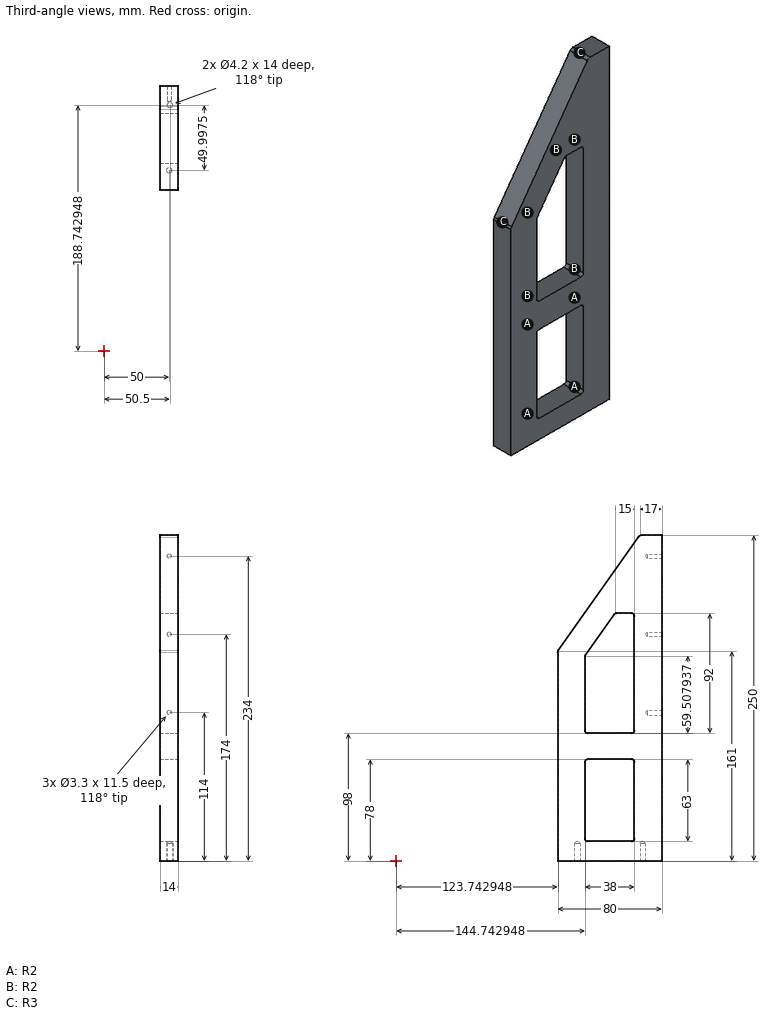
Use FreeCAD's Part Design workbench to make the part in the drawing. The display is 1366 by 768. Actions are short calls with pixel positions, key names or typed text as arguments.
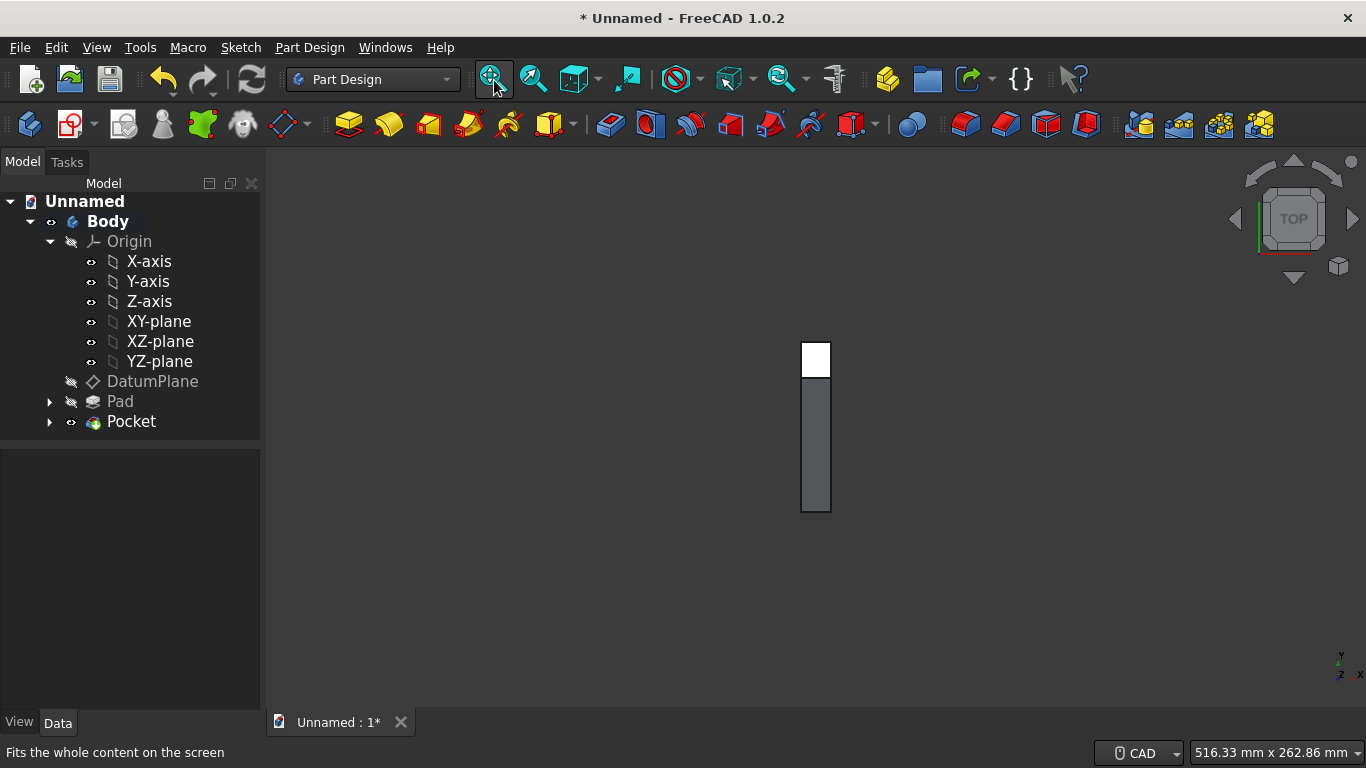
key(1)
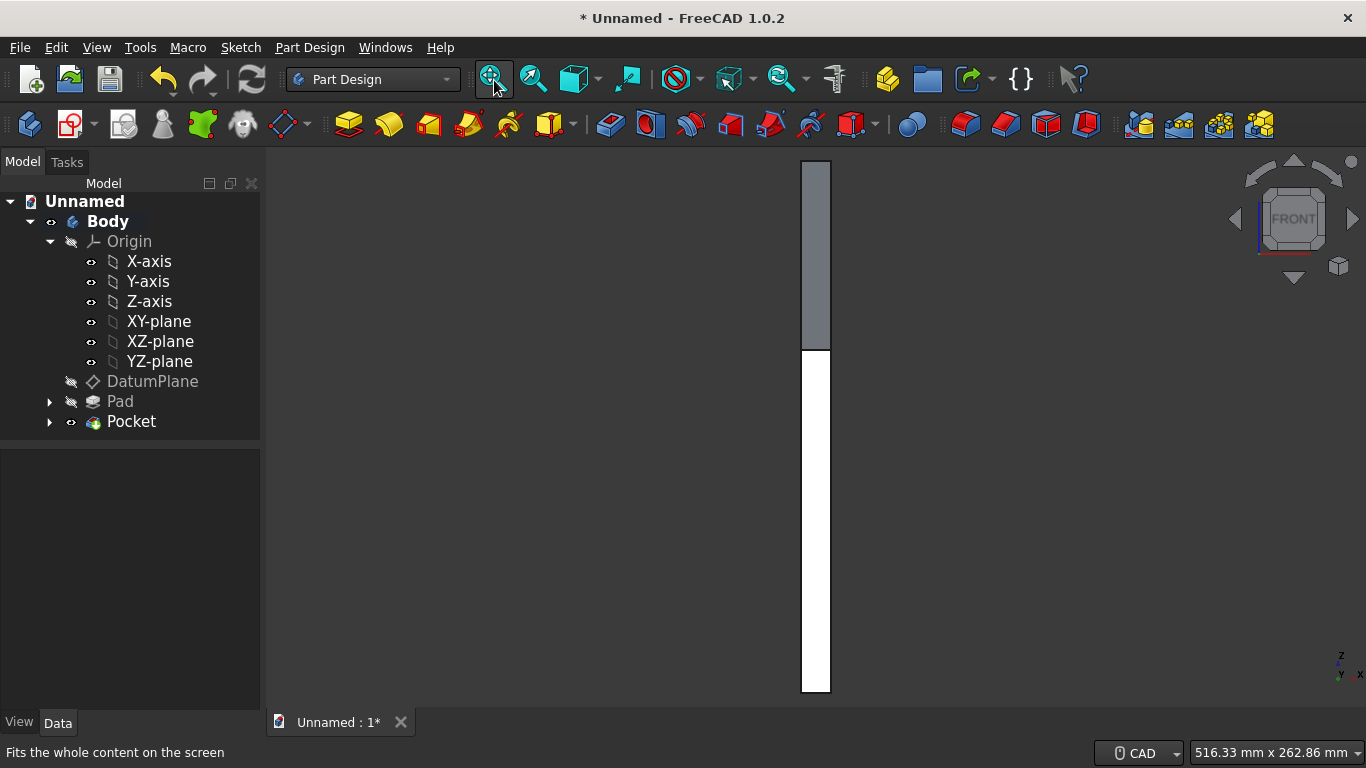
key(3)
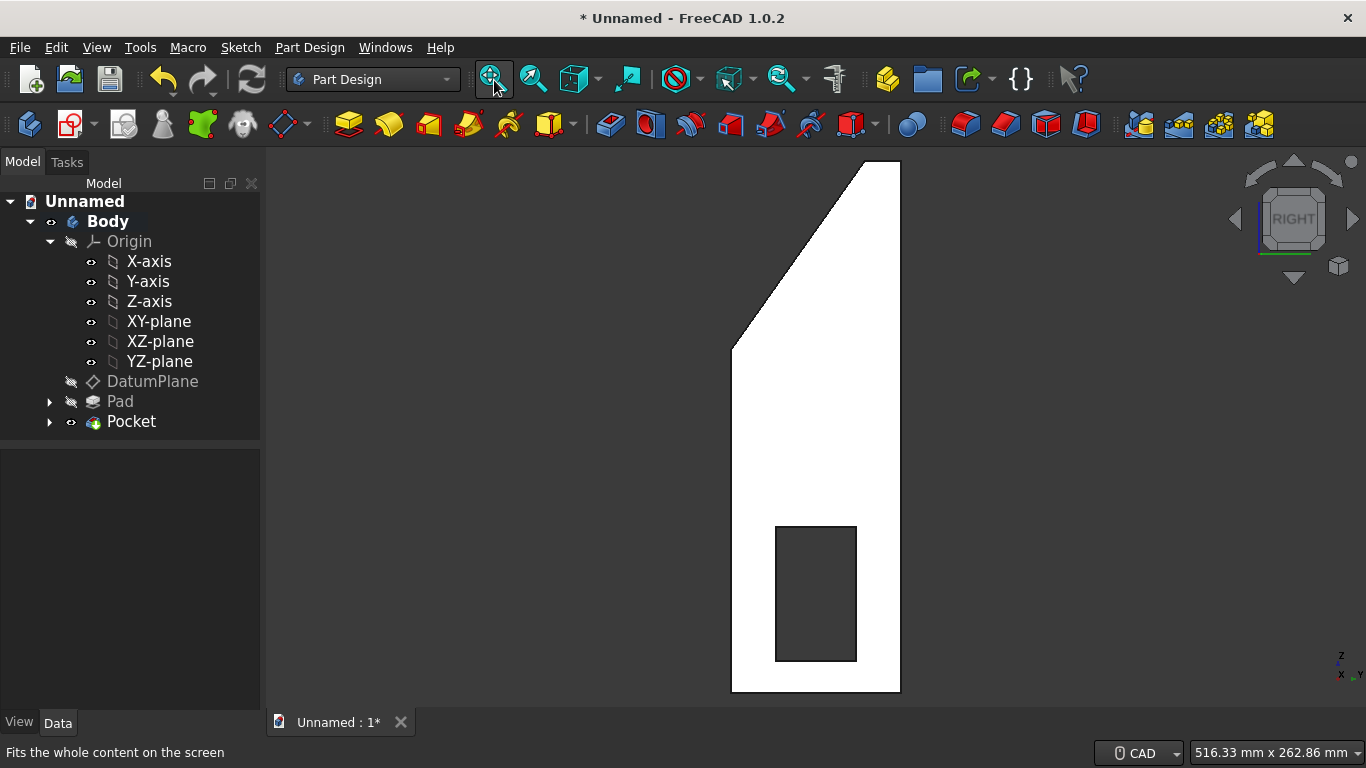
key(5)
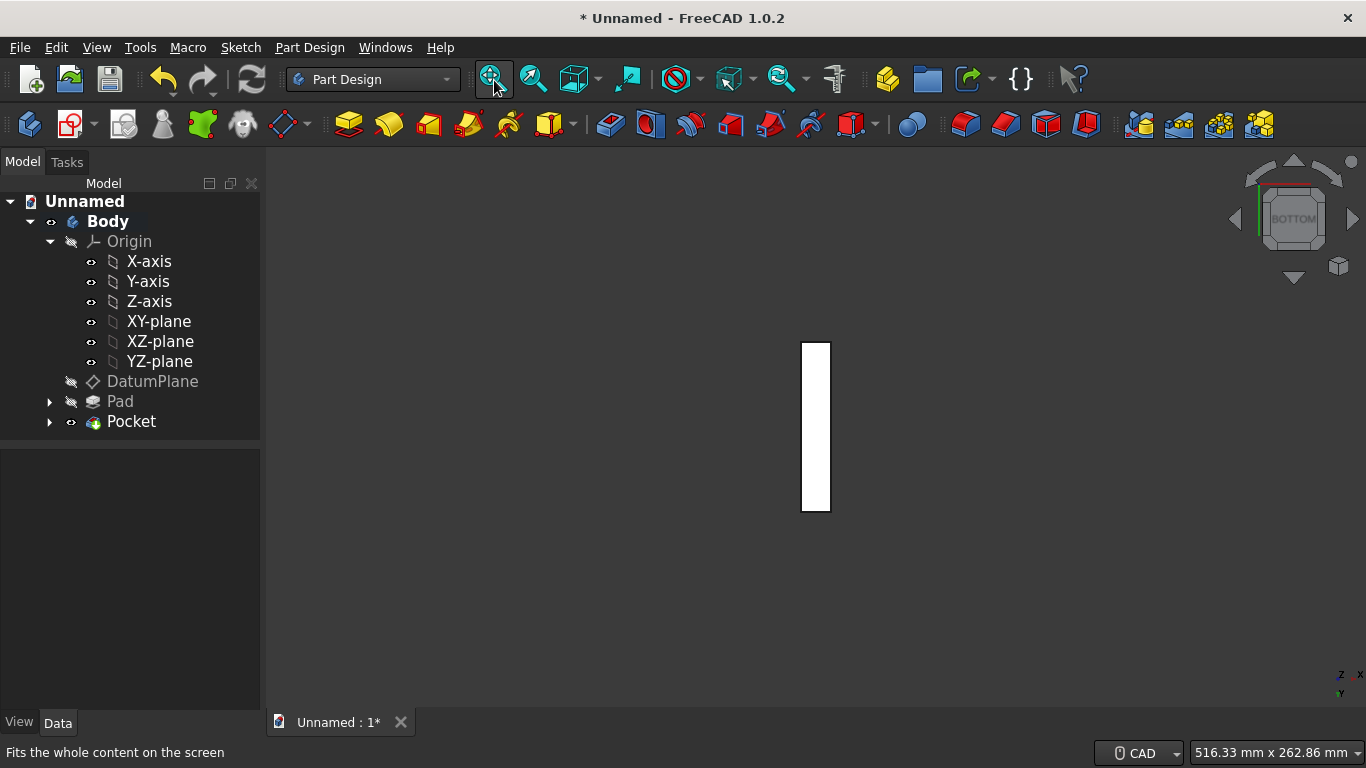
click(494, 80)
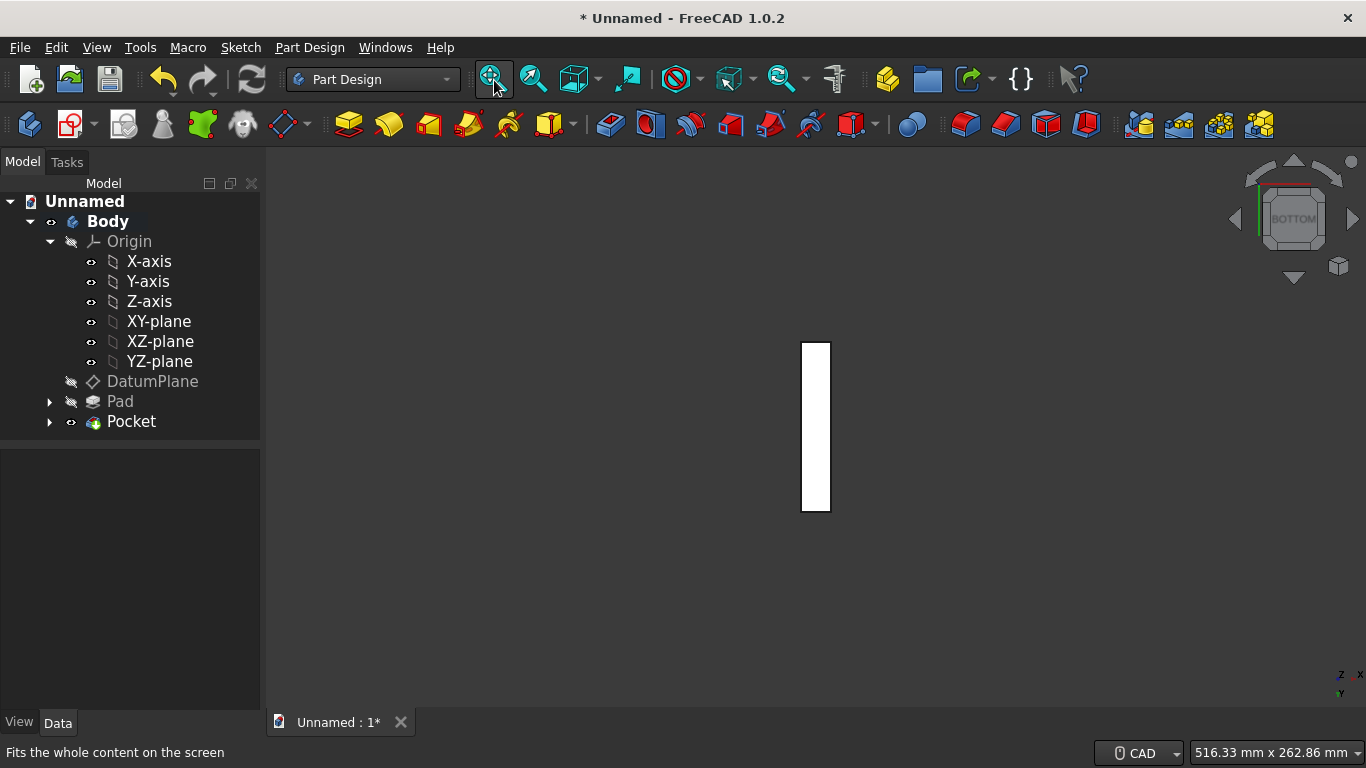
key(4)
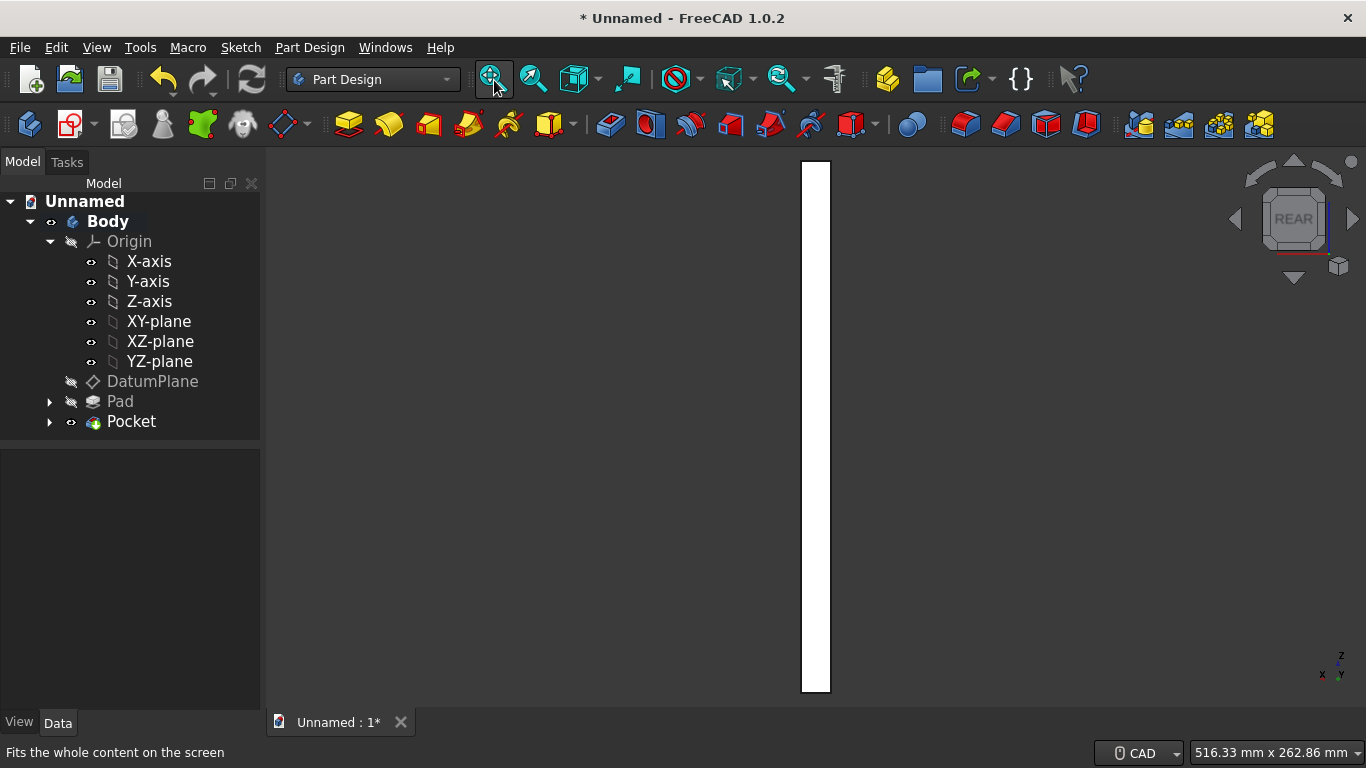
key(6)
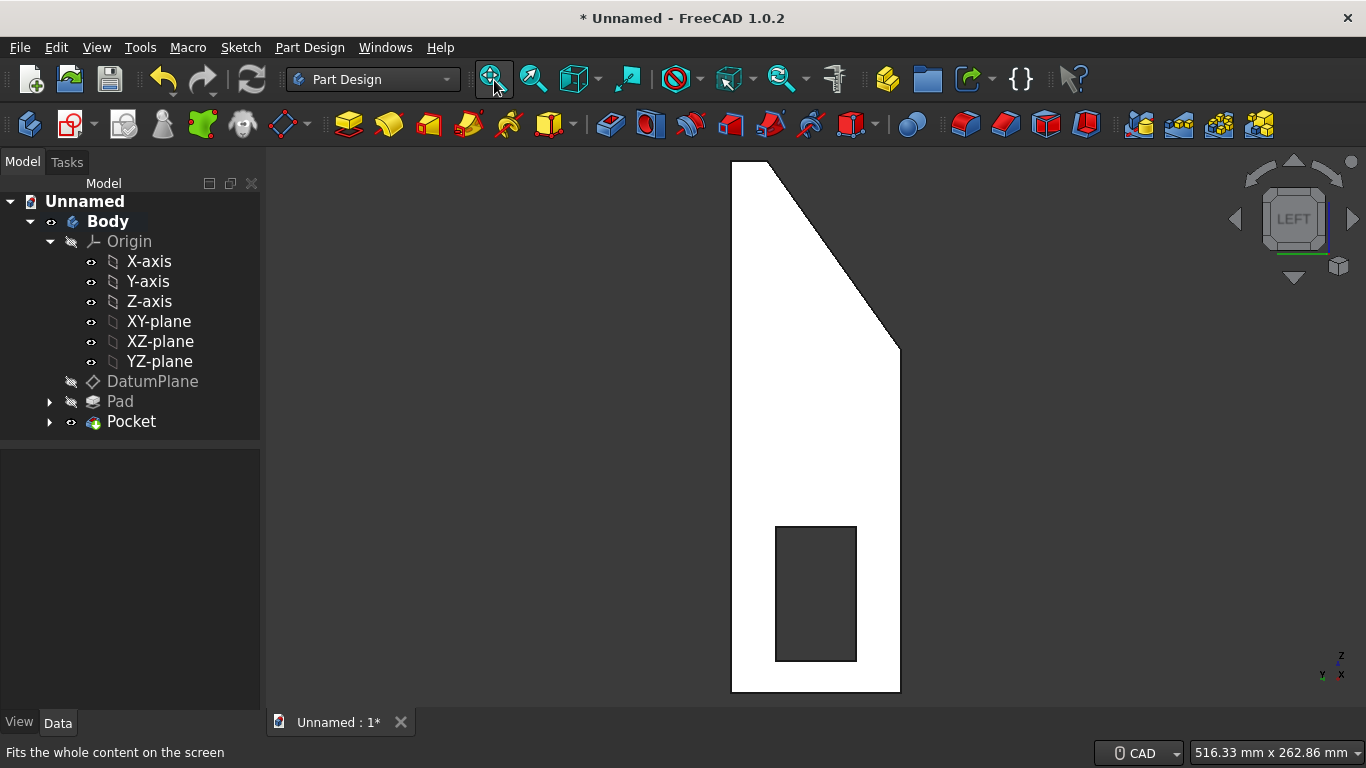
key(v)
key(3)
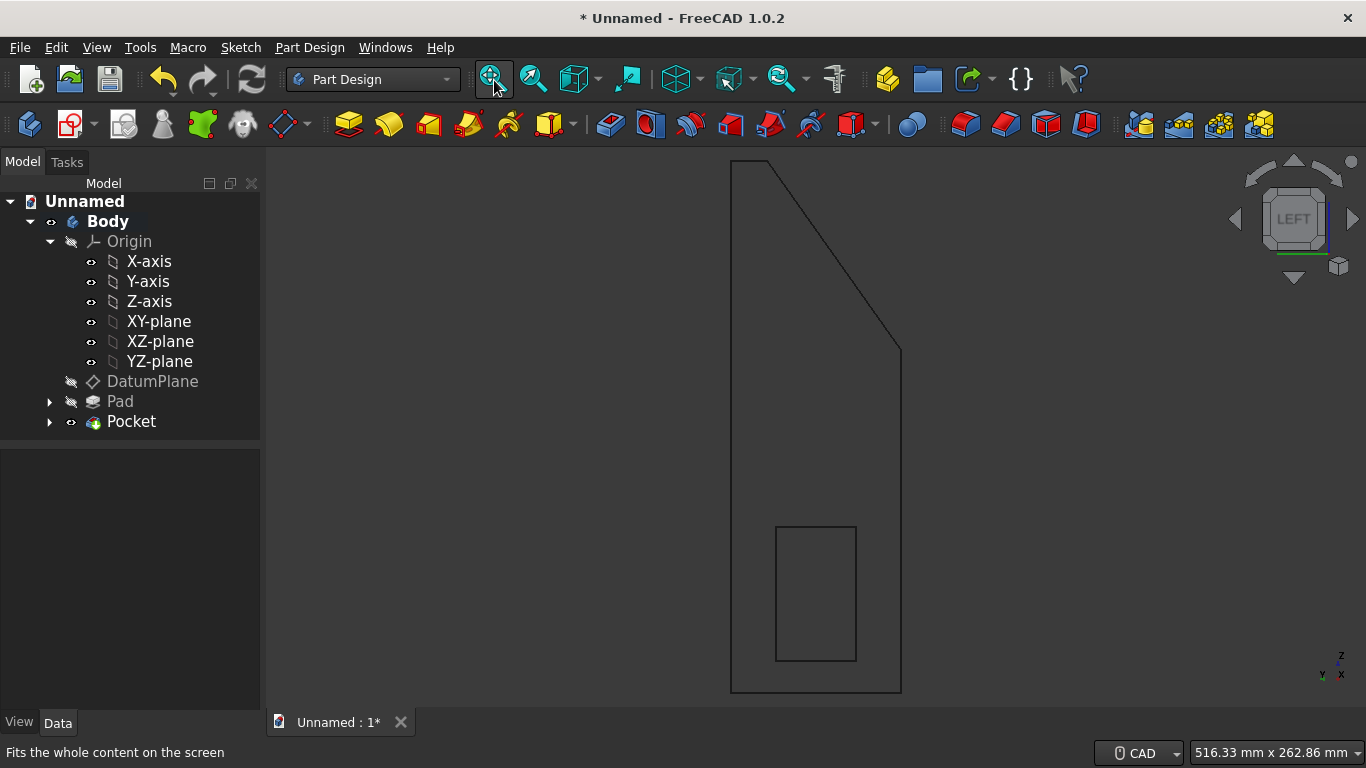
key(0)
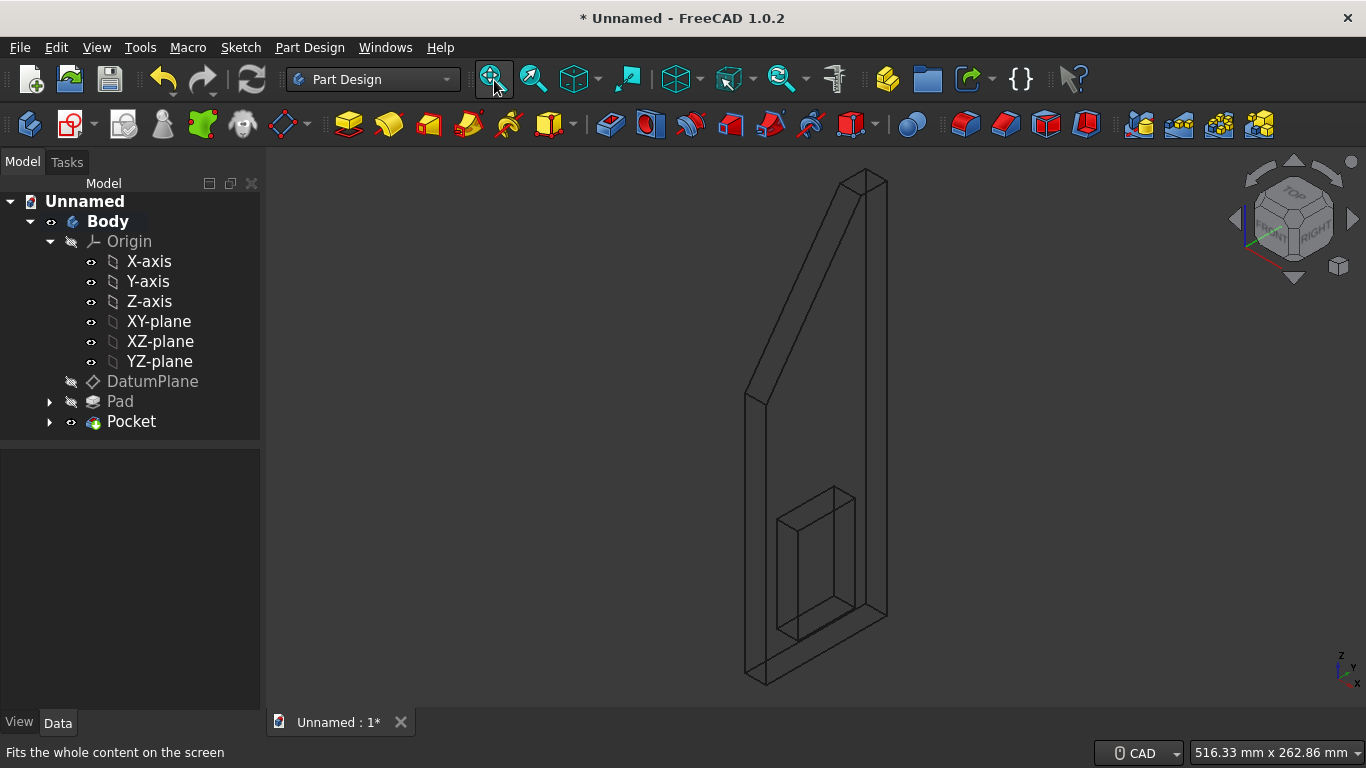
click(845, 601)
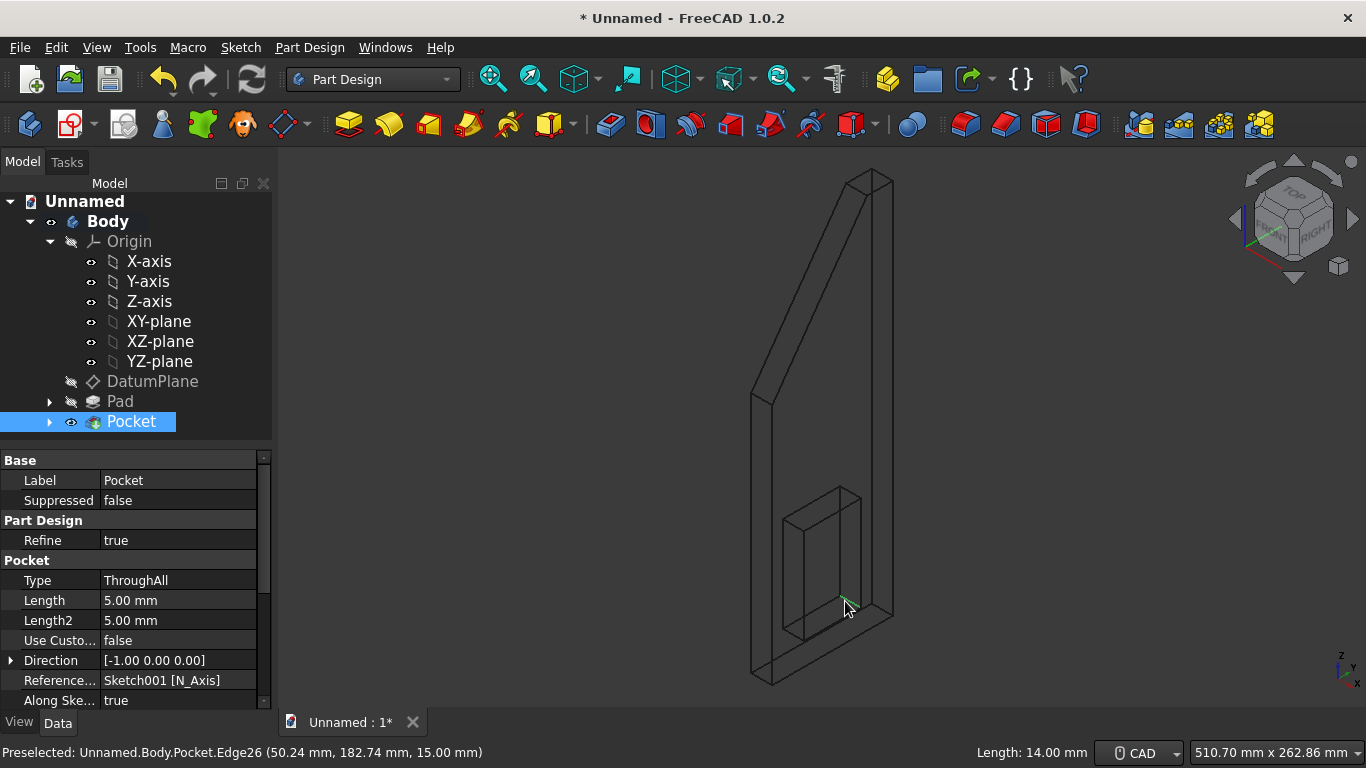
click(793, 634, ctrl)